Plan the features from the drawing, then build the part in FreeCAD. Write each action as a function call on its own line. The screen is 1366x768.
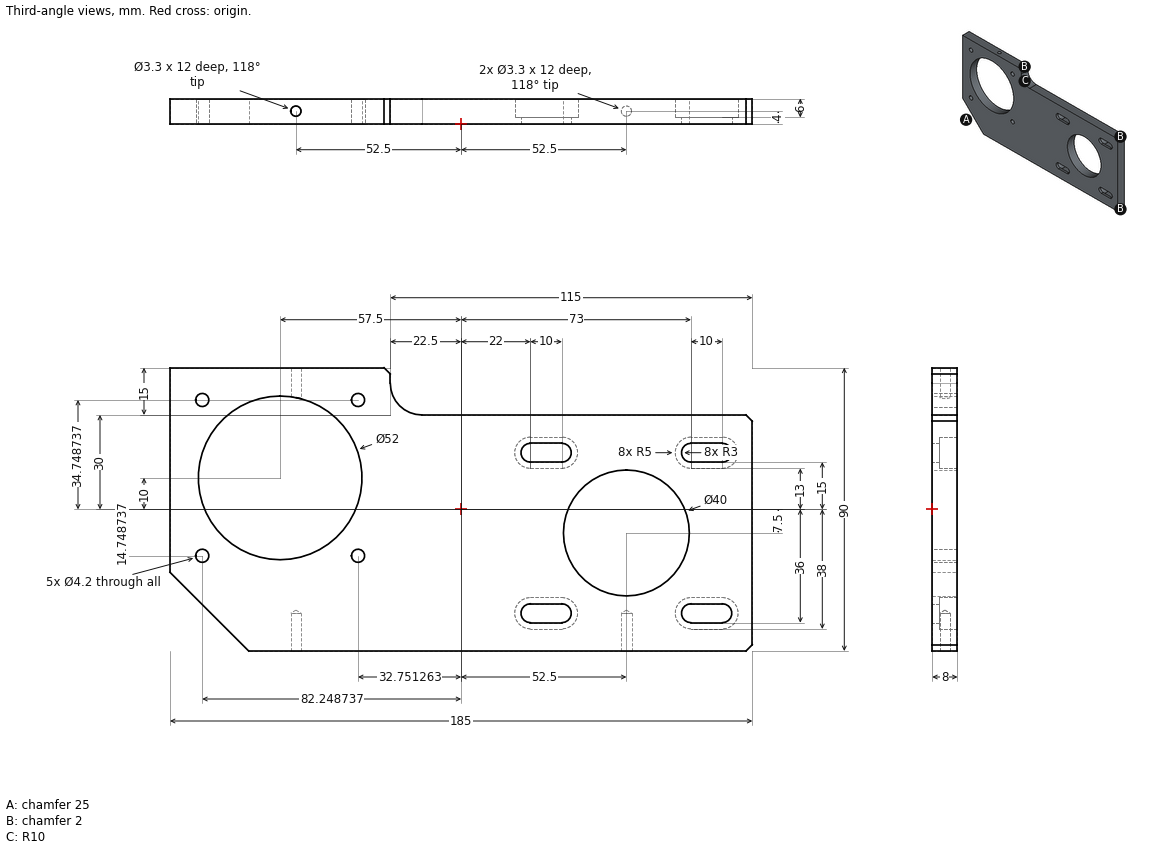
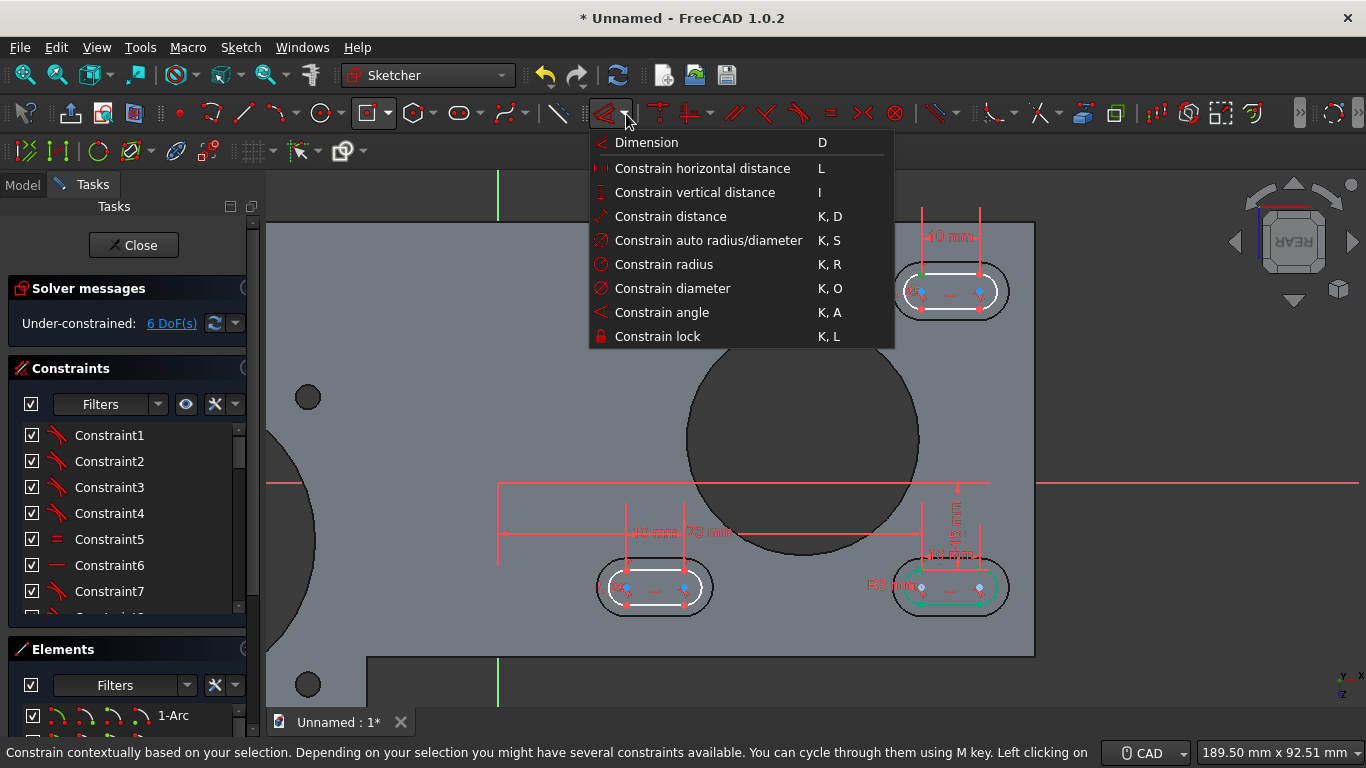
click(742, 168)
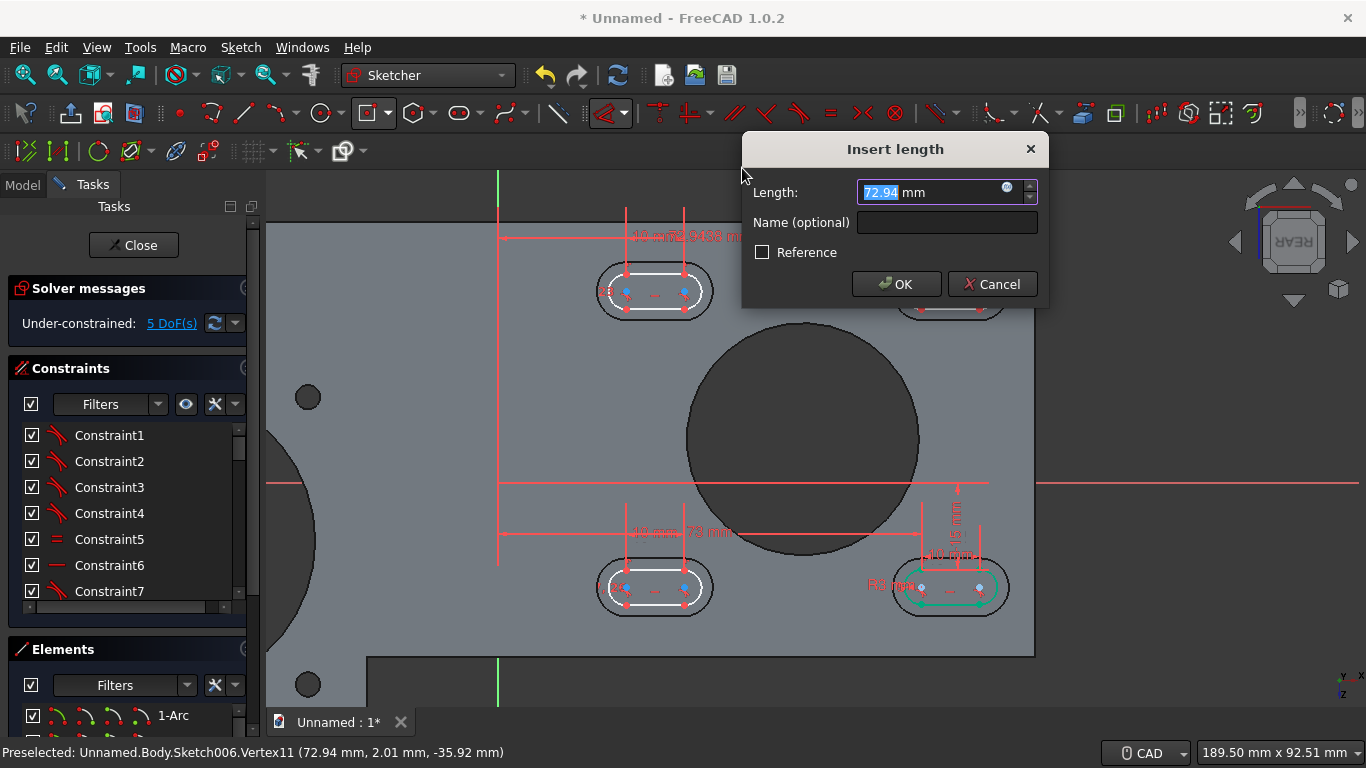
text(73)
key(Return)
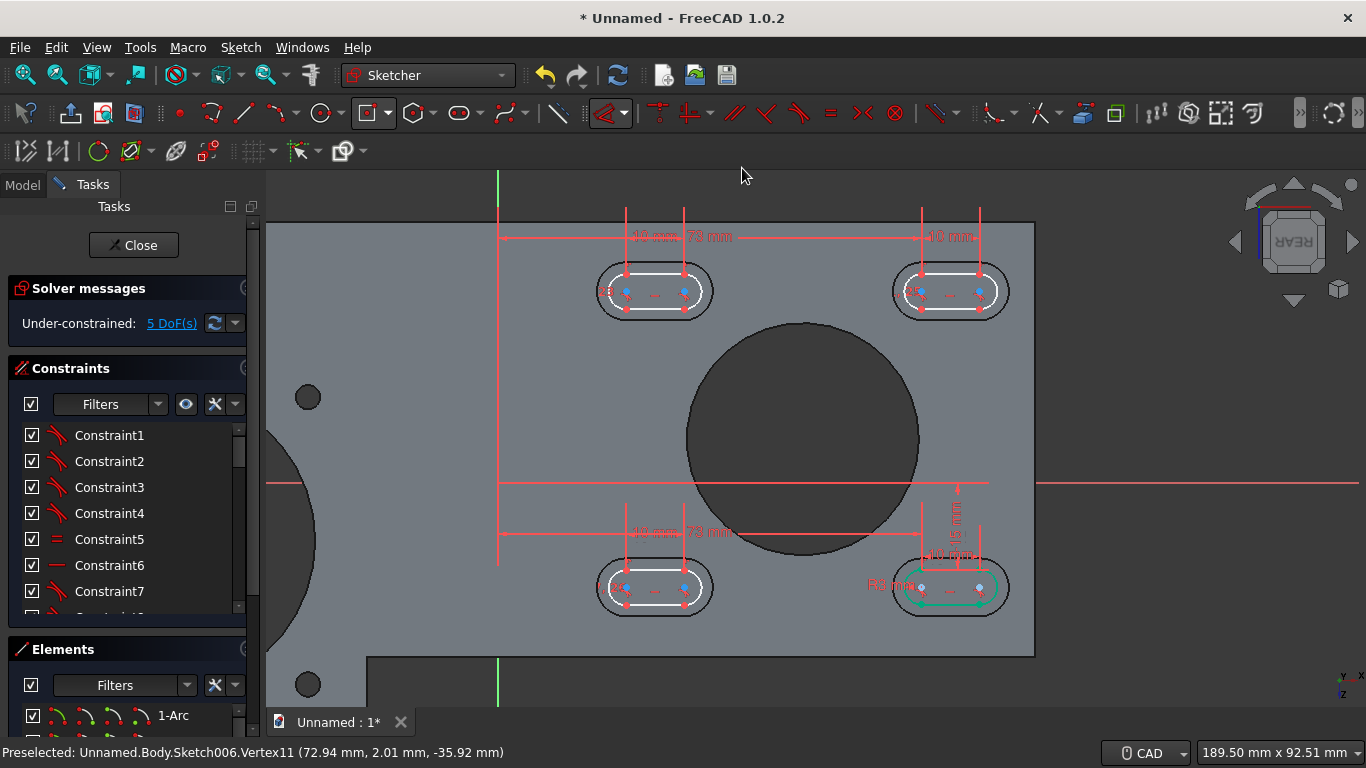
click(922, 274)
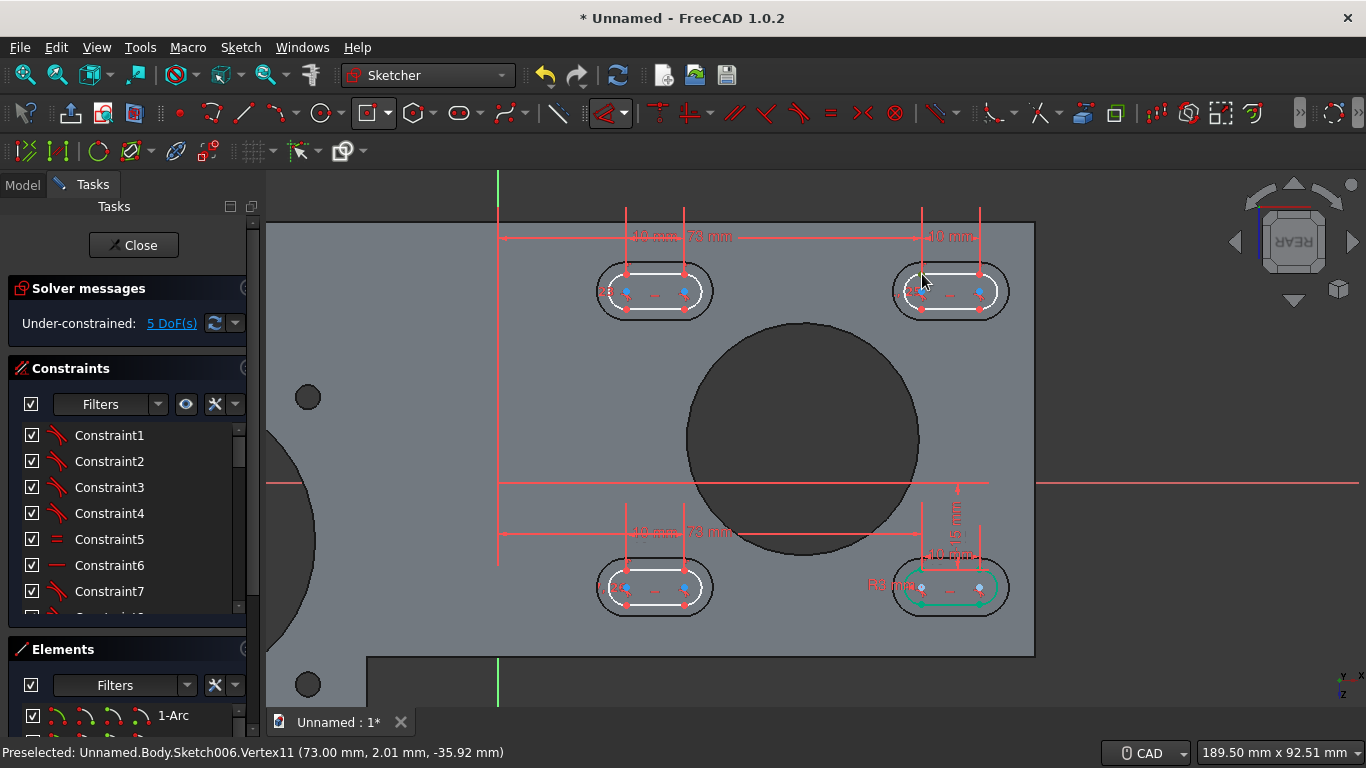
click(626, 114)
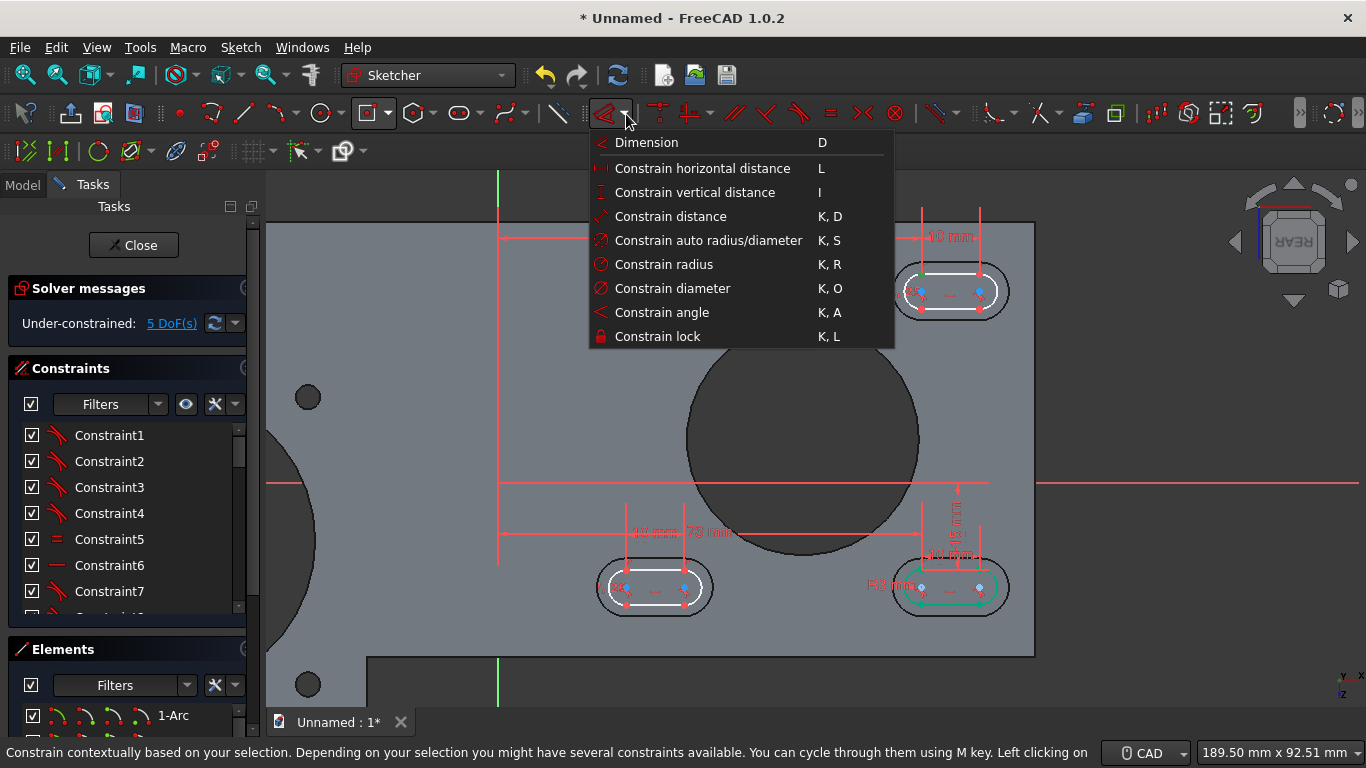
click(742, 192)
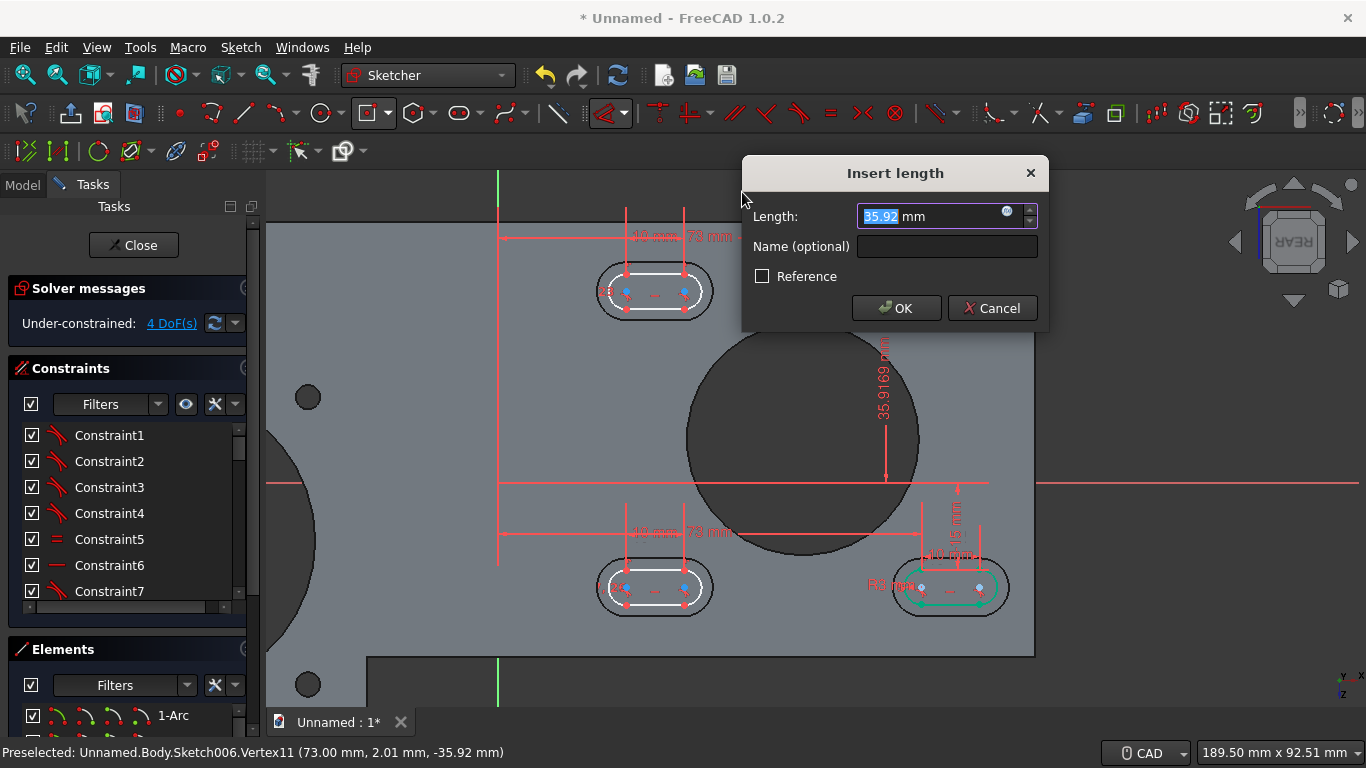
text(36)
key(Return)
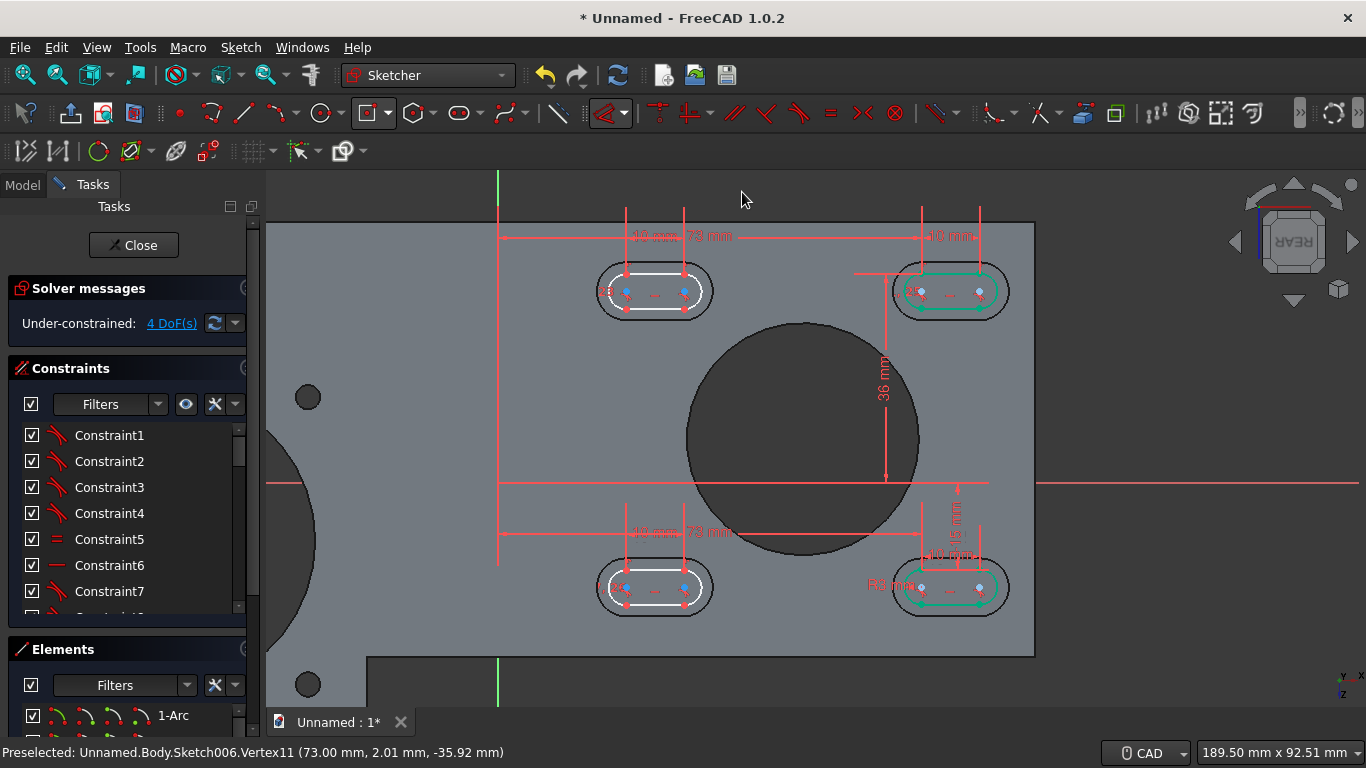
click(626, 570)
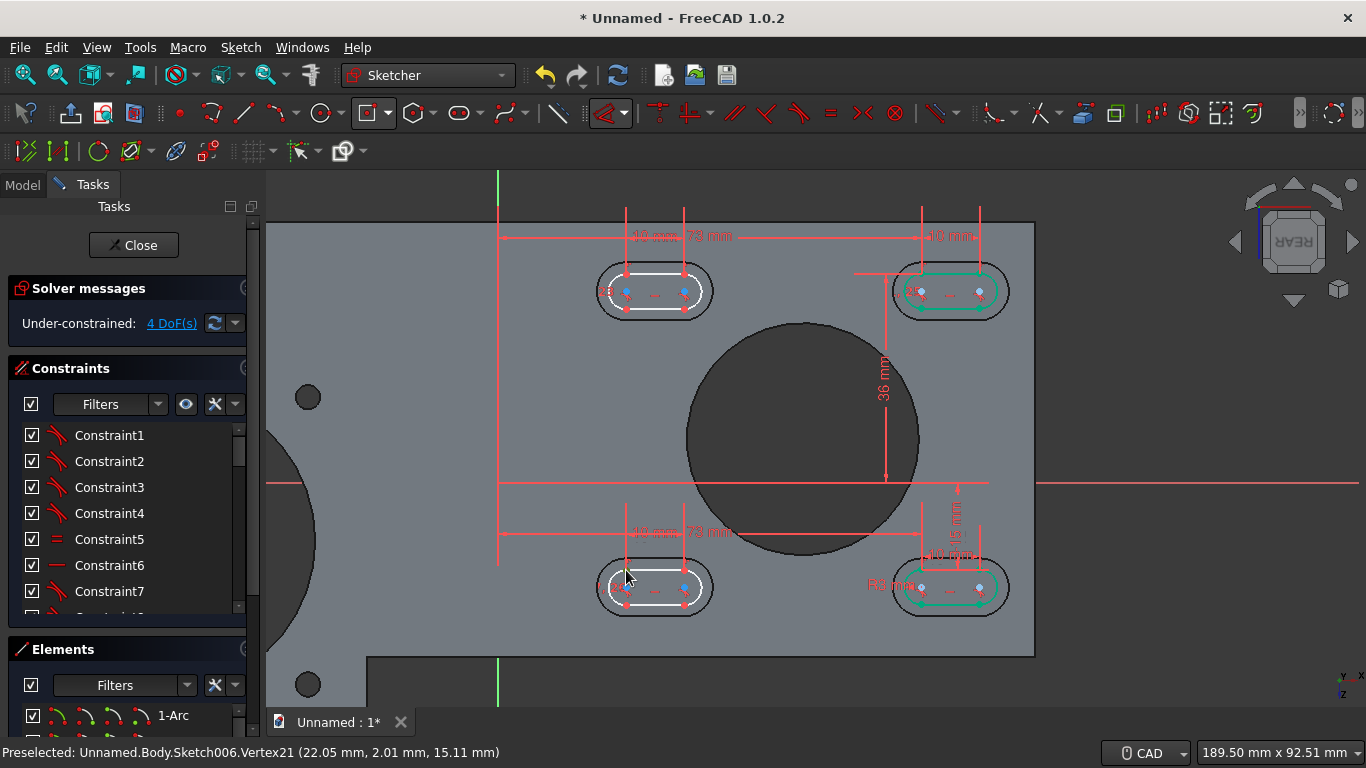
click(626, 114)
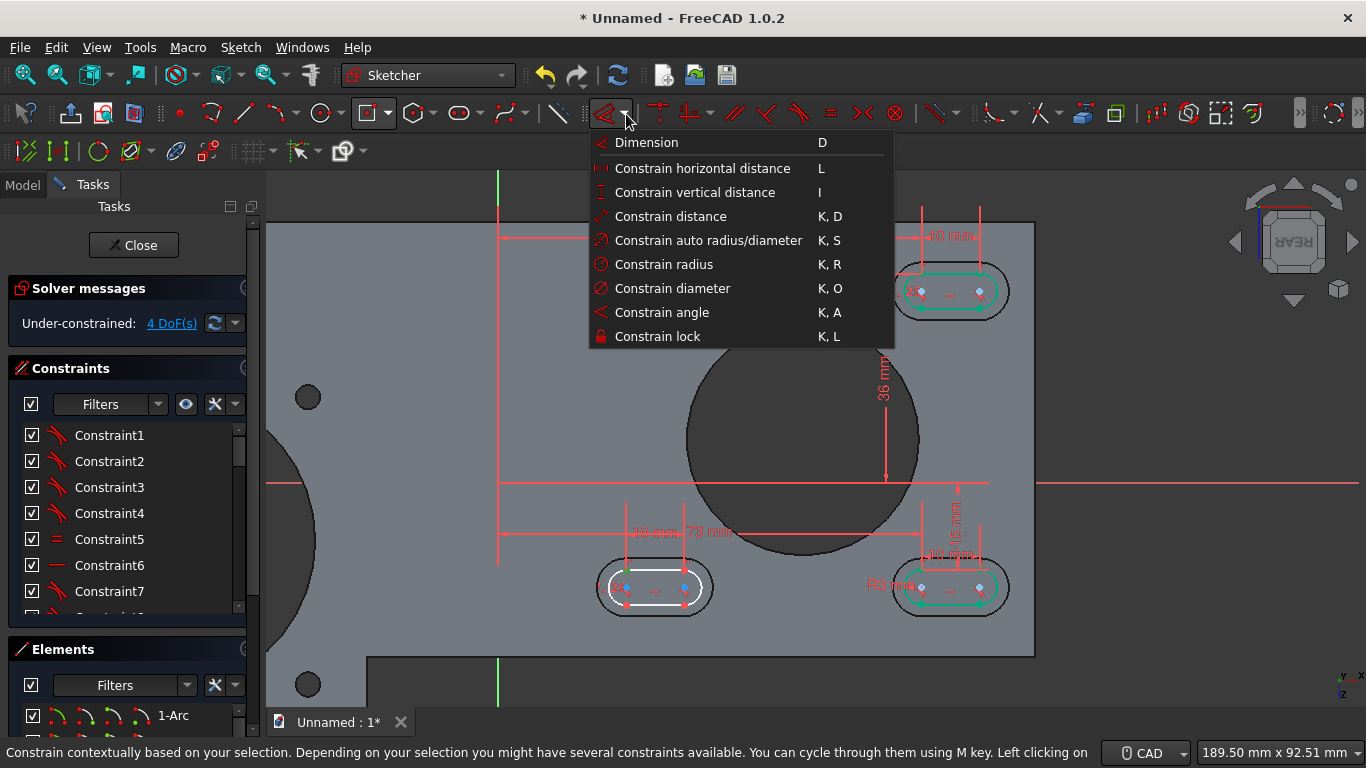
click(742, 168)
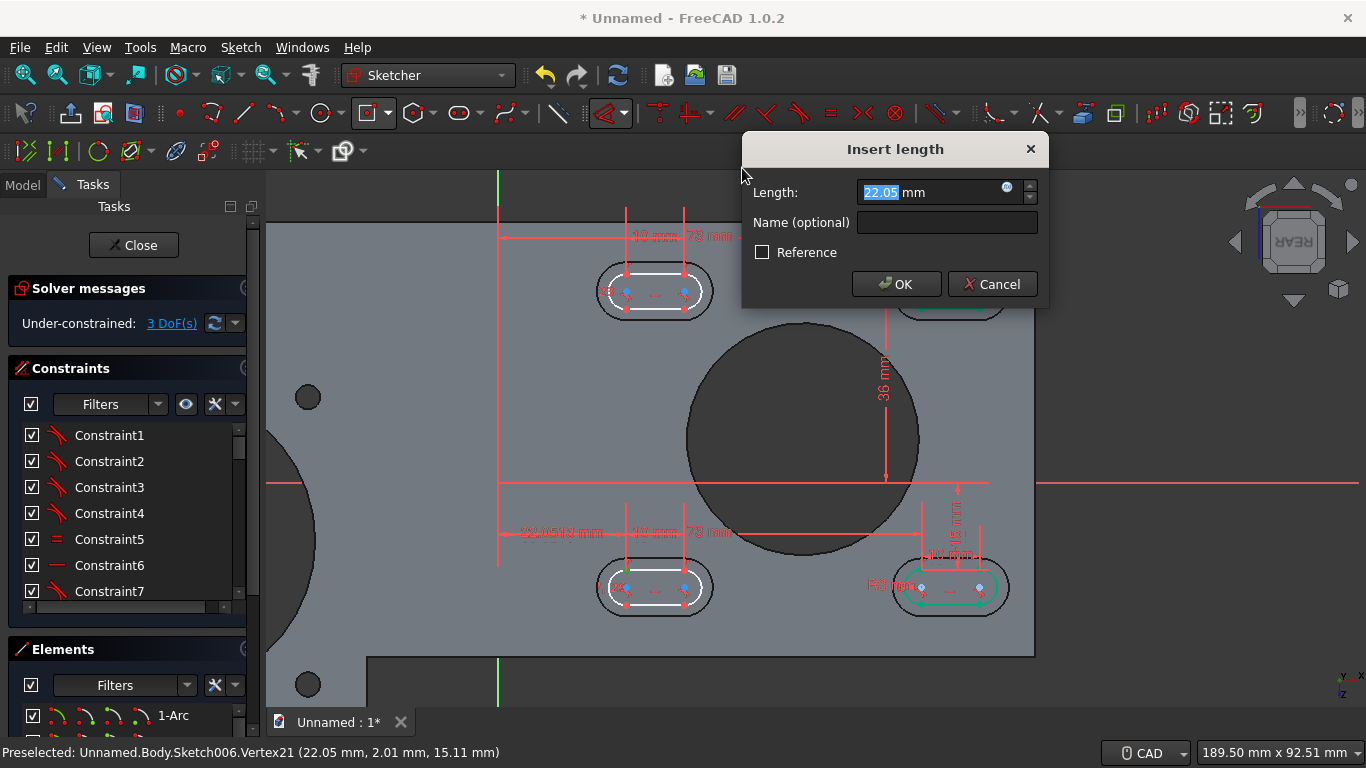
text(22)
key(Return)